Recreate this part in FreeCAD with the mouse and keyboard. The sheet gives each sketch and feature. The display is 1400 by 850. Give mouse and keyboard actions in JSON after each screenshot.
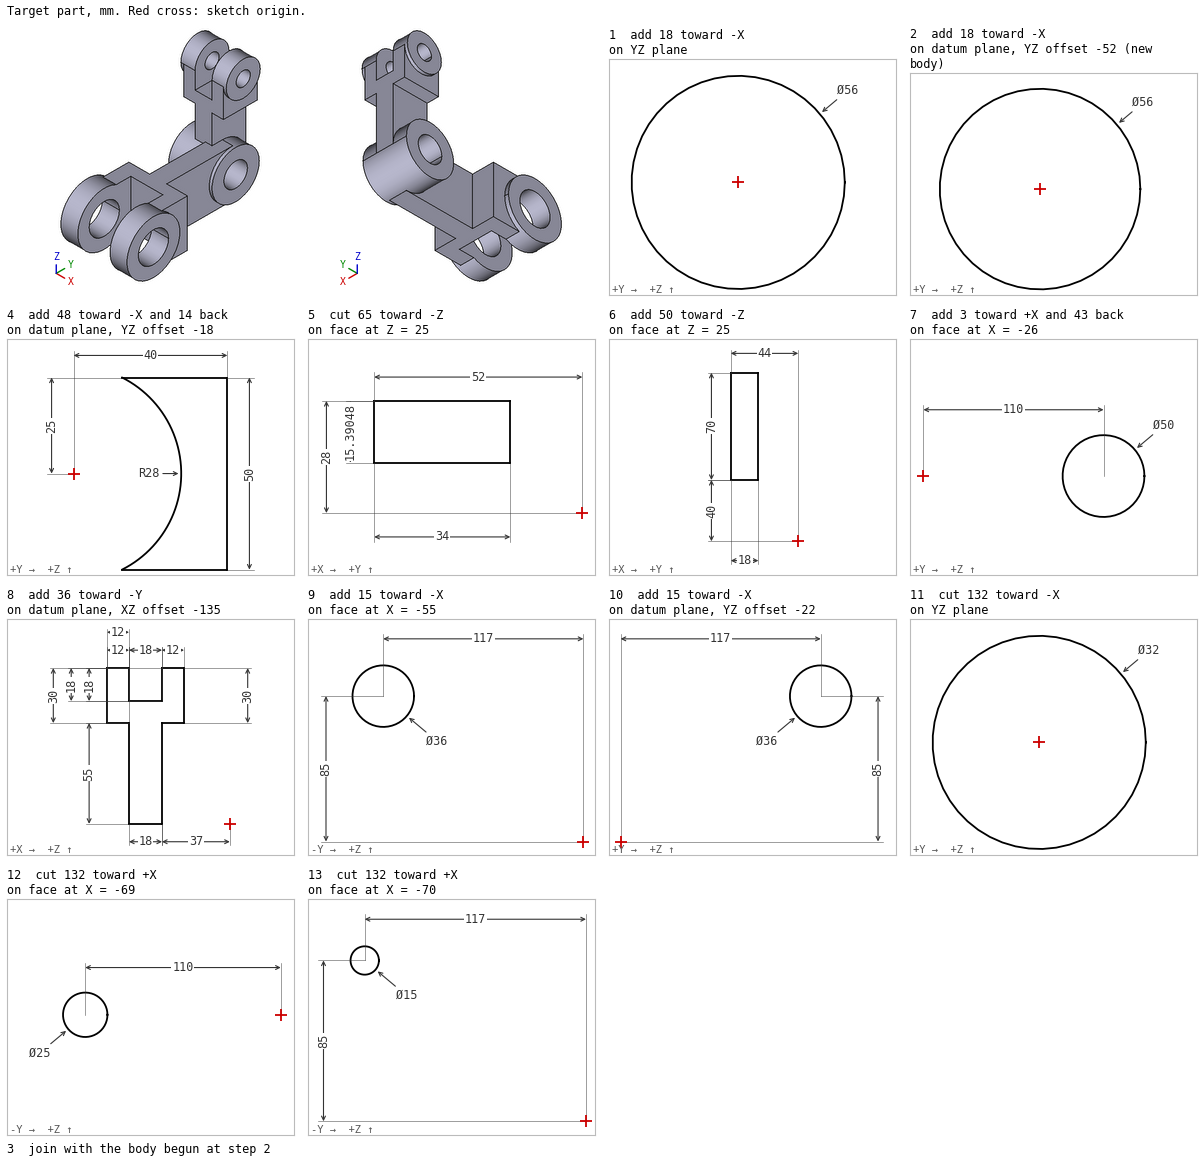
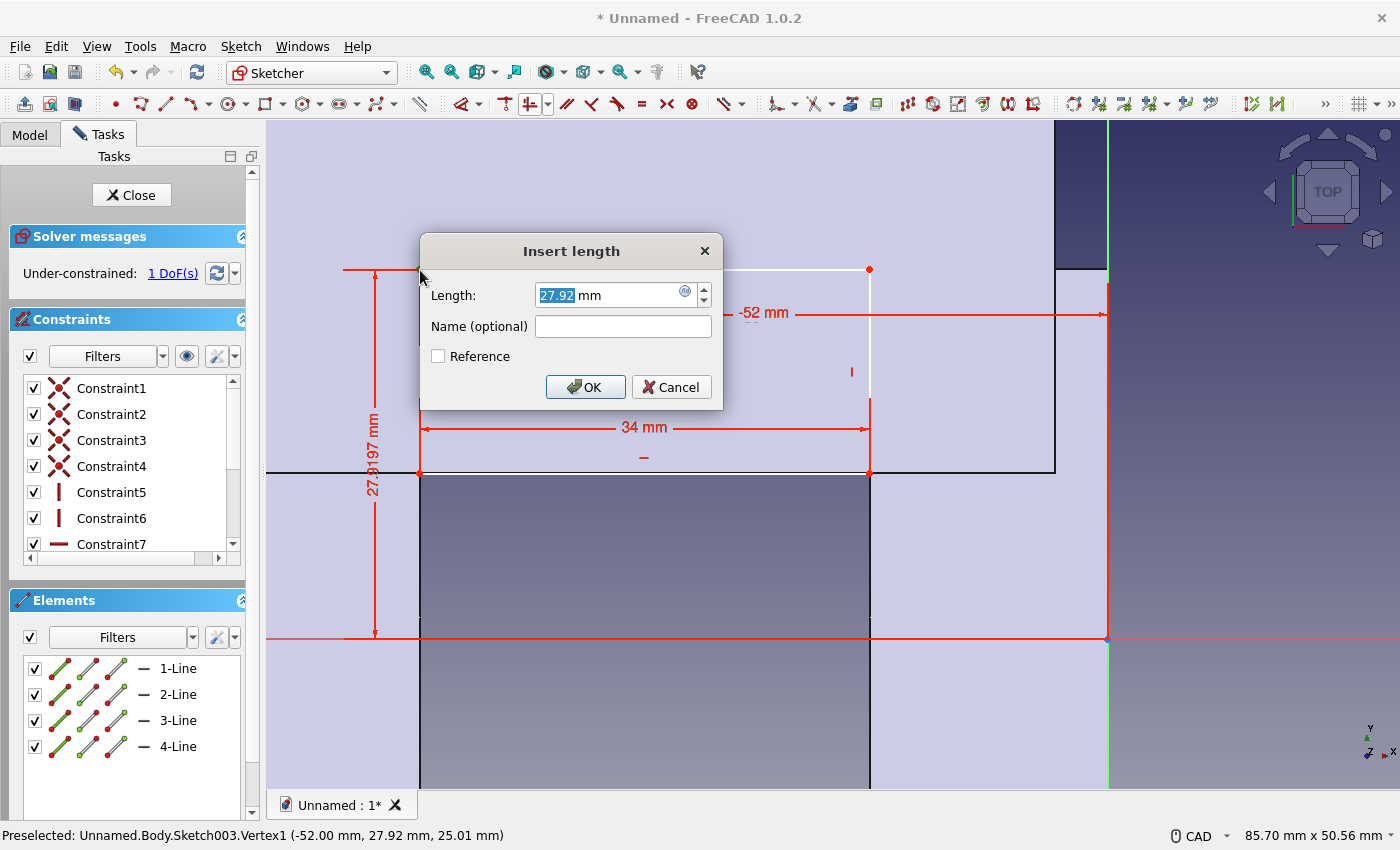
{"action": "type", "text": "28"}
{"action": "key", "text": "Return"}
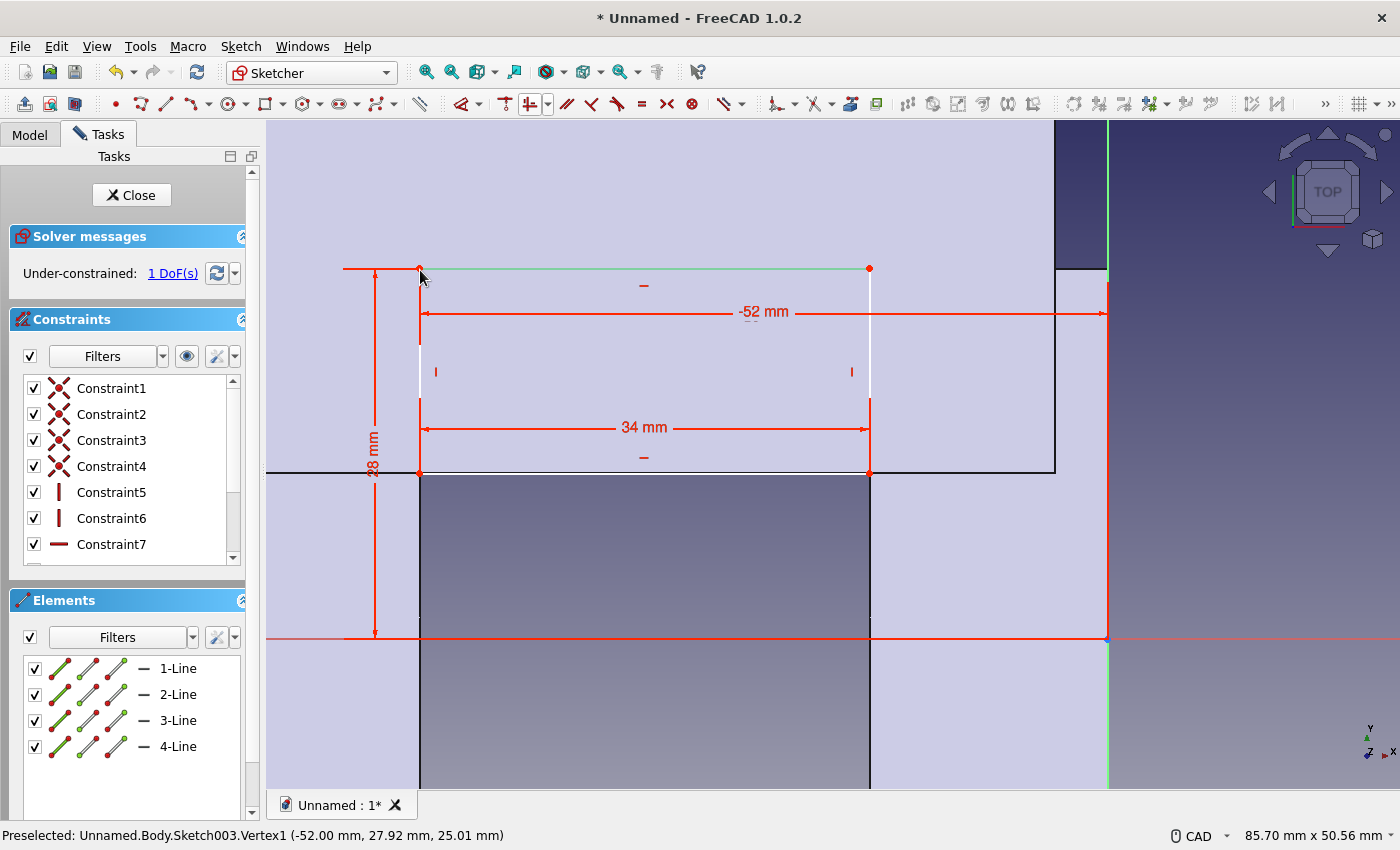
{"action": "left_click", "coordinate": [420, 330]}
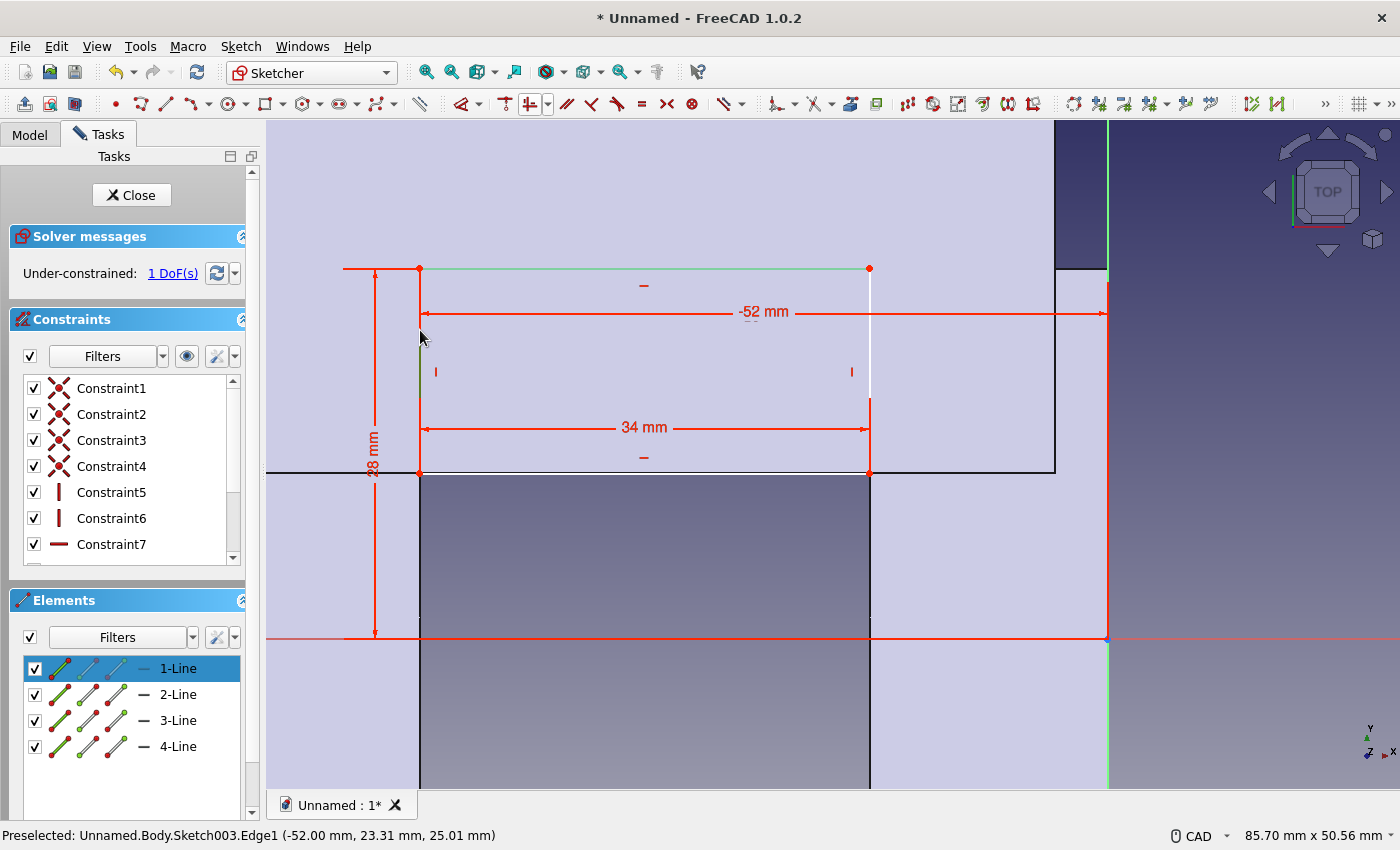
{"action": "key", "text": "i"}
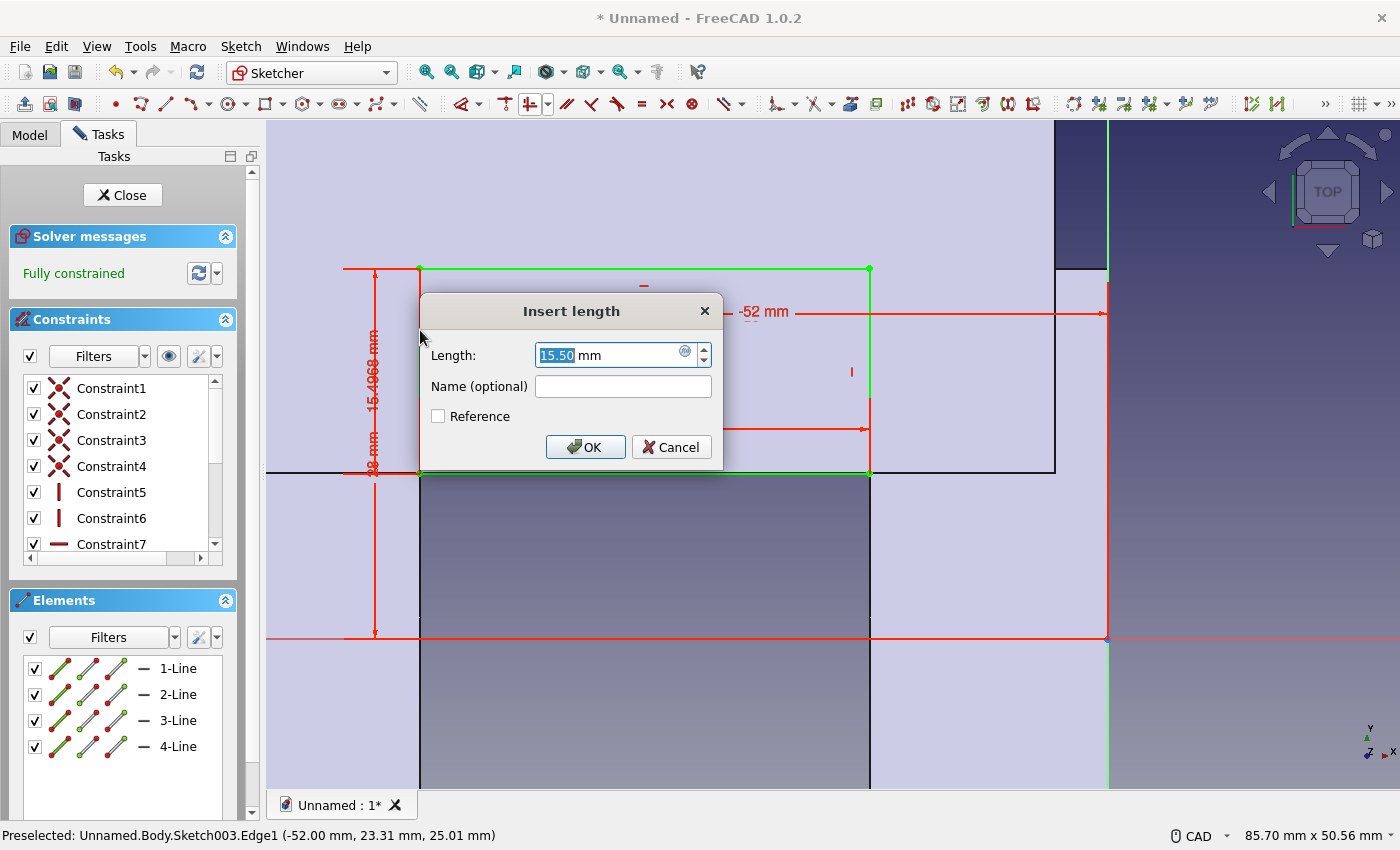
{"action": "type", "text": "15.39048"}
{"action": "key", "text": "Return"}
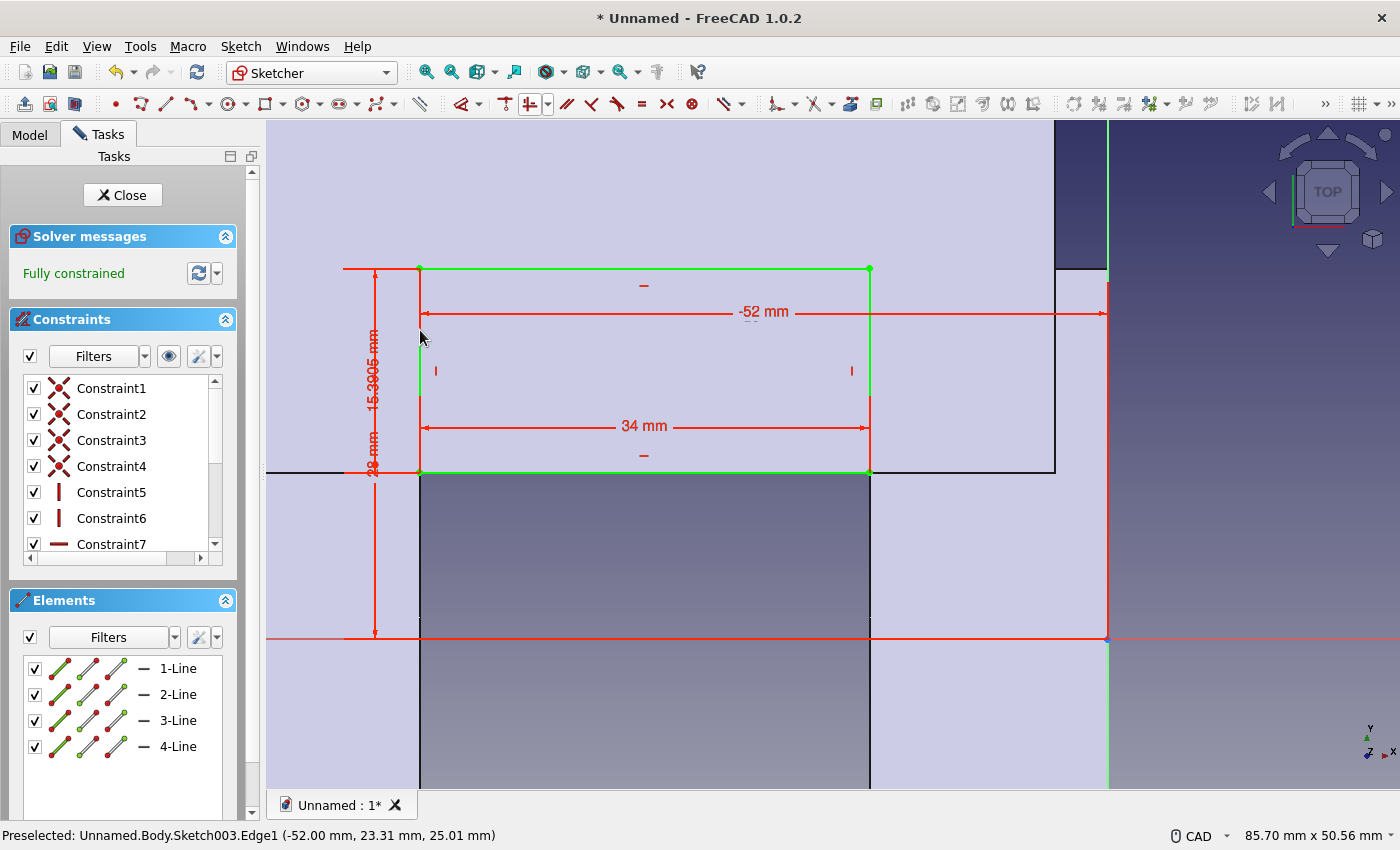
{"action": "left_click", "coordinate": [123, 195]}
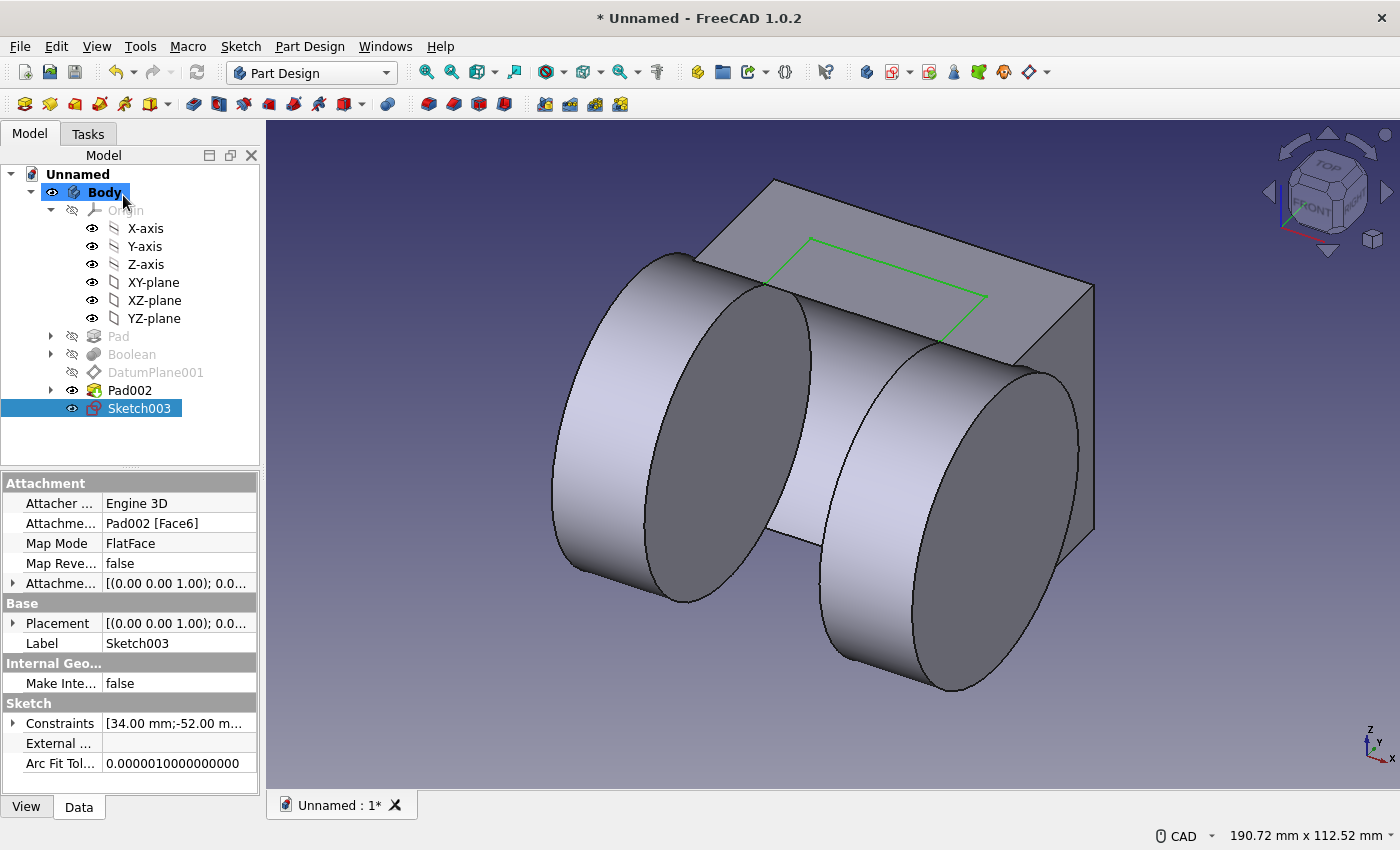
{"action": "left_click", "coordinate": [194, 104]}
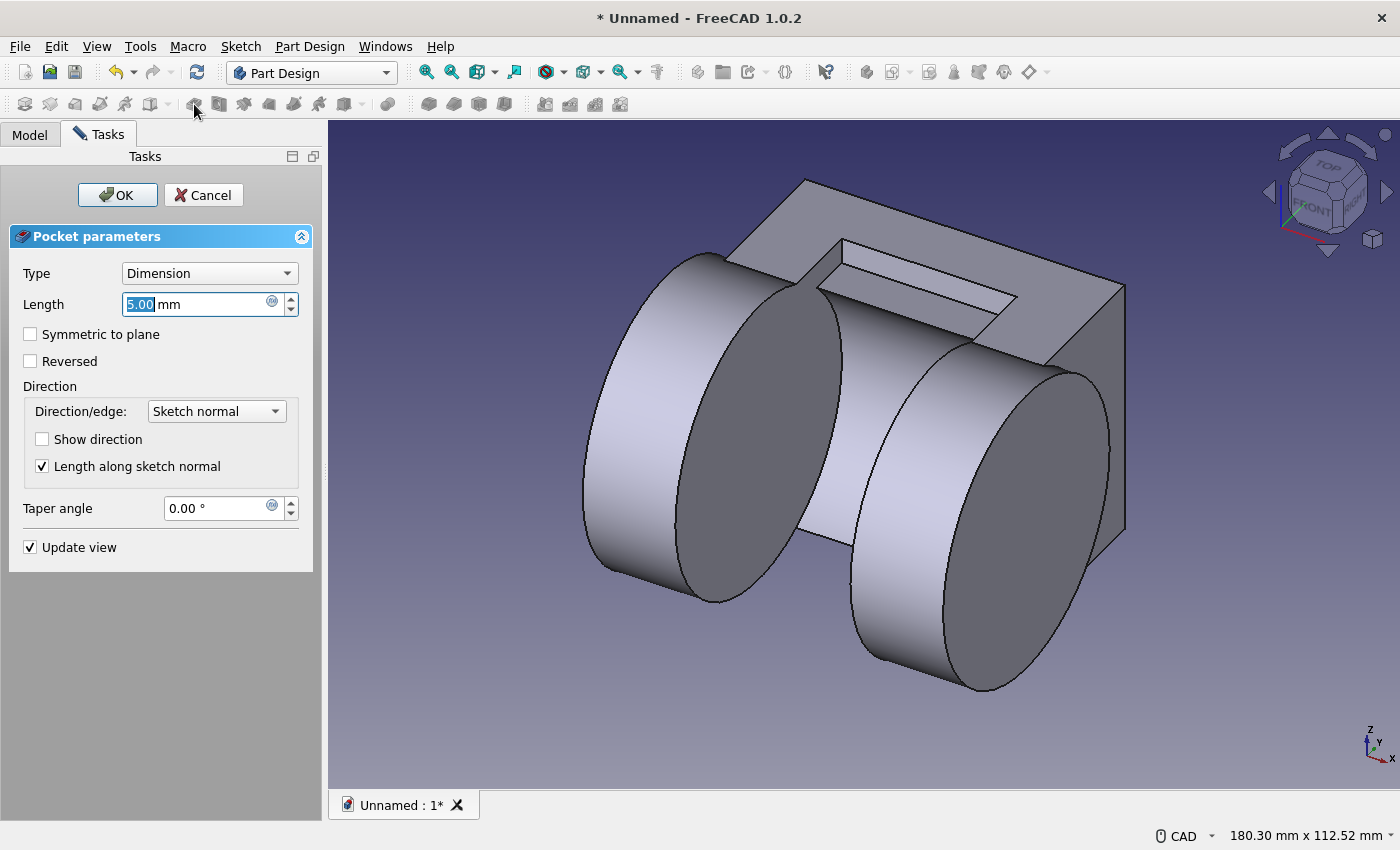
{"action": "type", "text": "65"}
{"action": "key", "text": "Tab"}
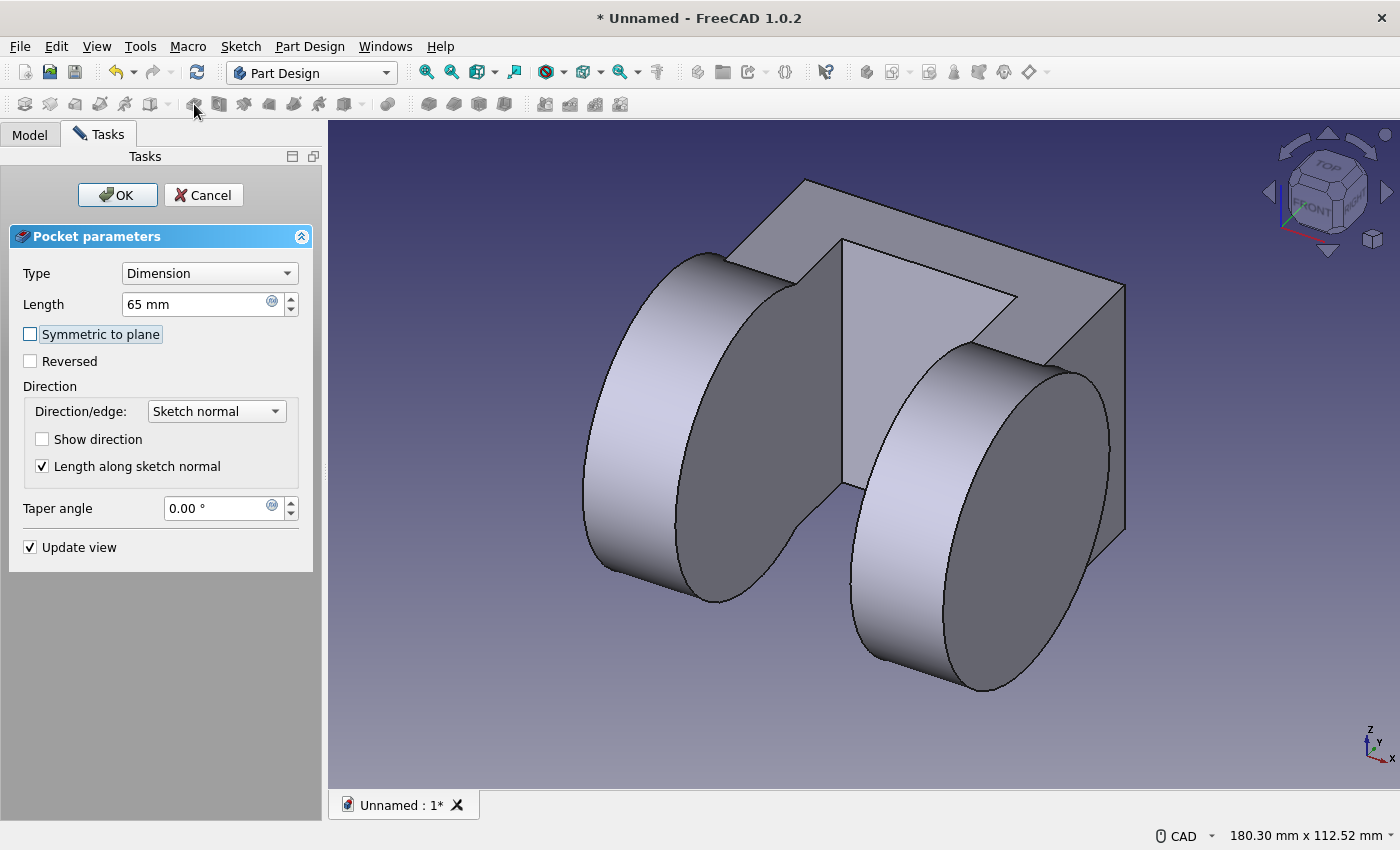
{"action": "left_click", "coordinate": [118, 195]}